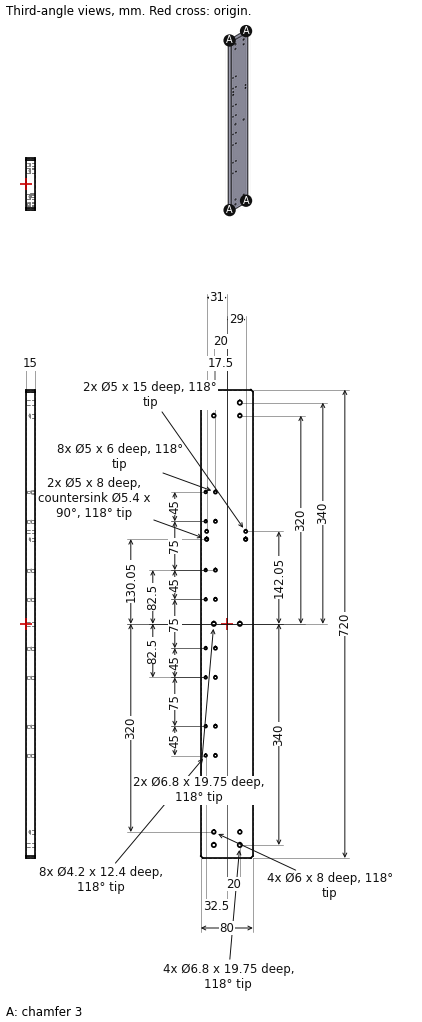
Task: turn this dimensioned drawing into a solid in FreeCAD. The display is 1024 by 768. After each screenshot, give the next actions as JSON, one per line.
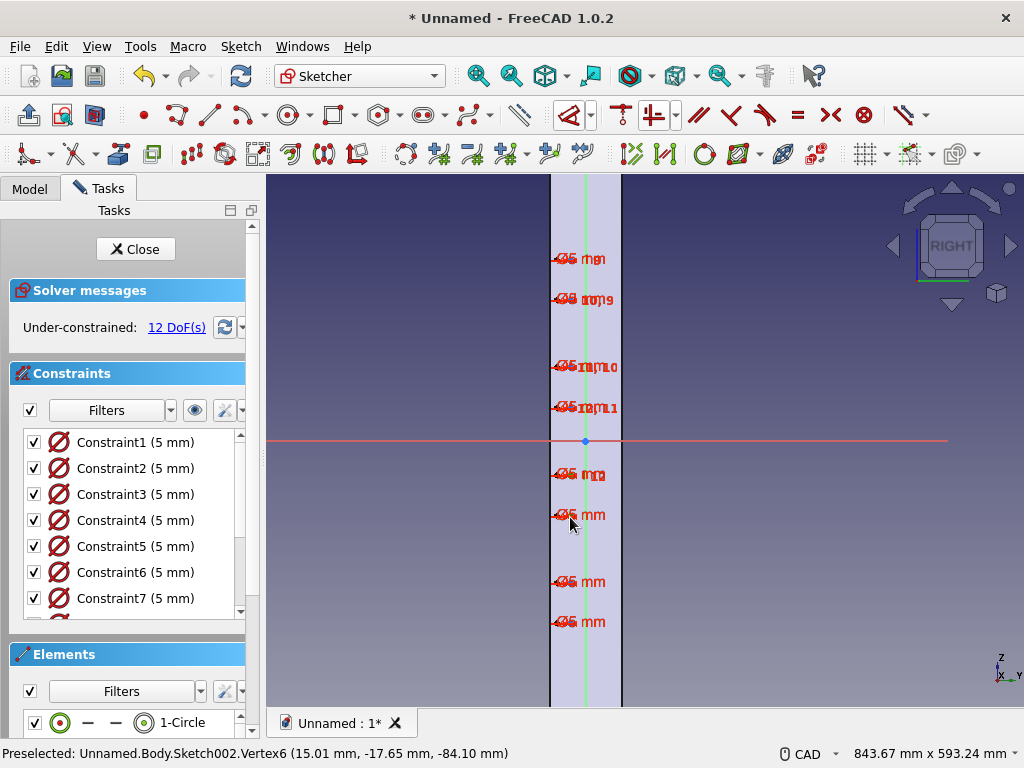
{"action": "left_click", "coordinate": [676, 116]}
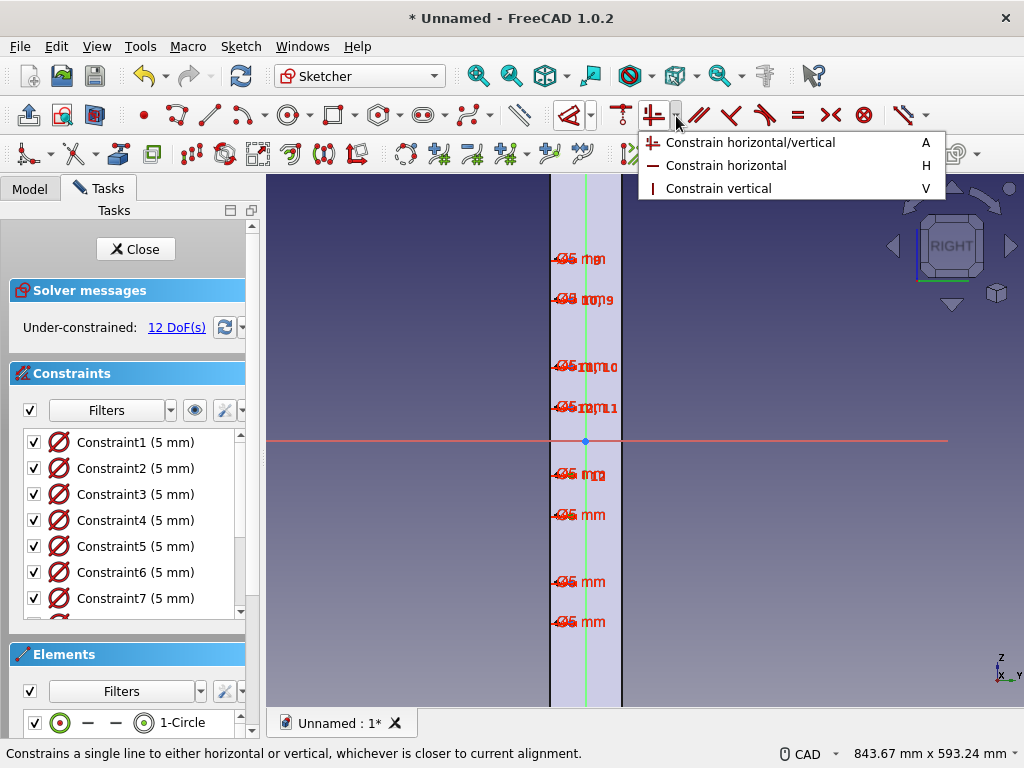
{"action": "left_click", "coordinate": [792, 188]}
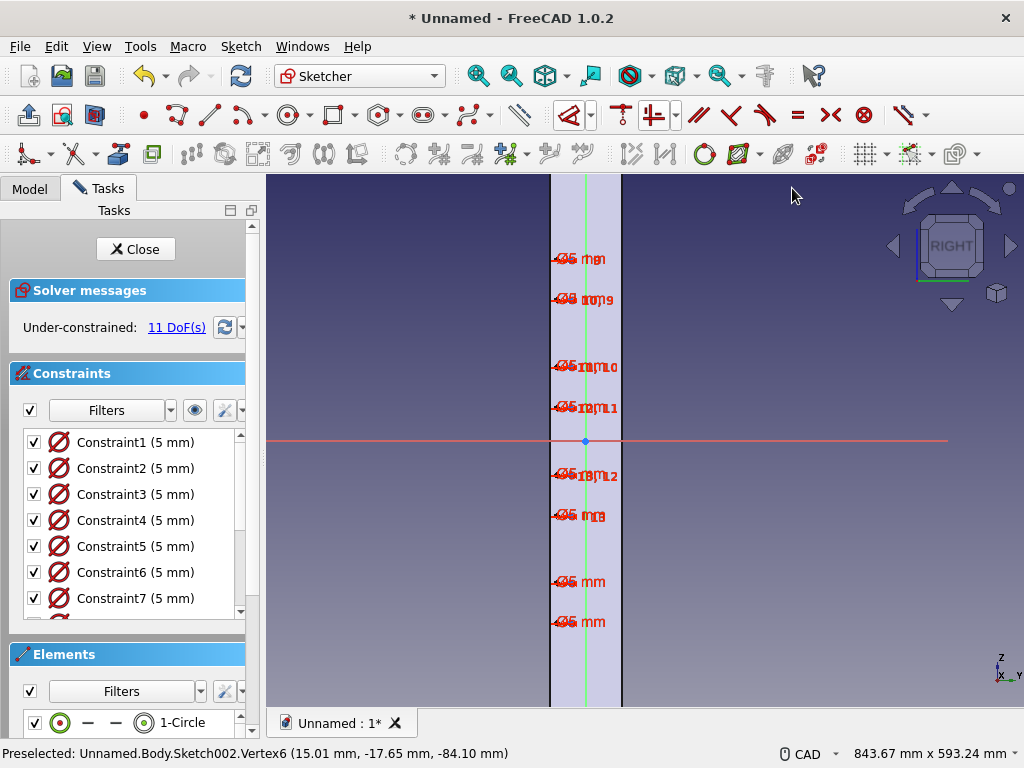
{"action": "left_click", "coordinate": [570, 517]}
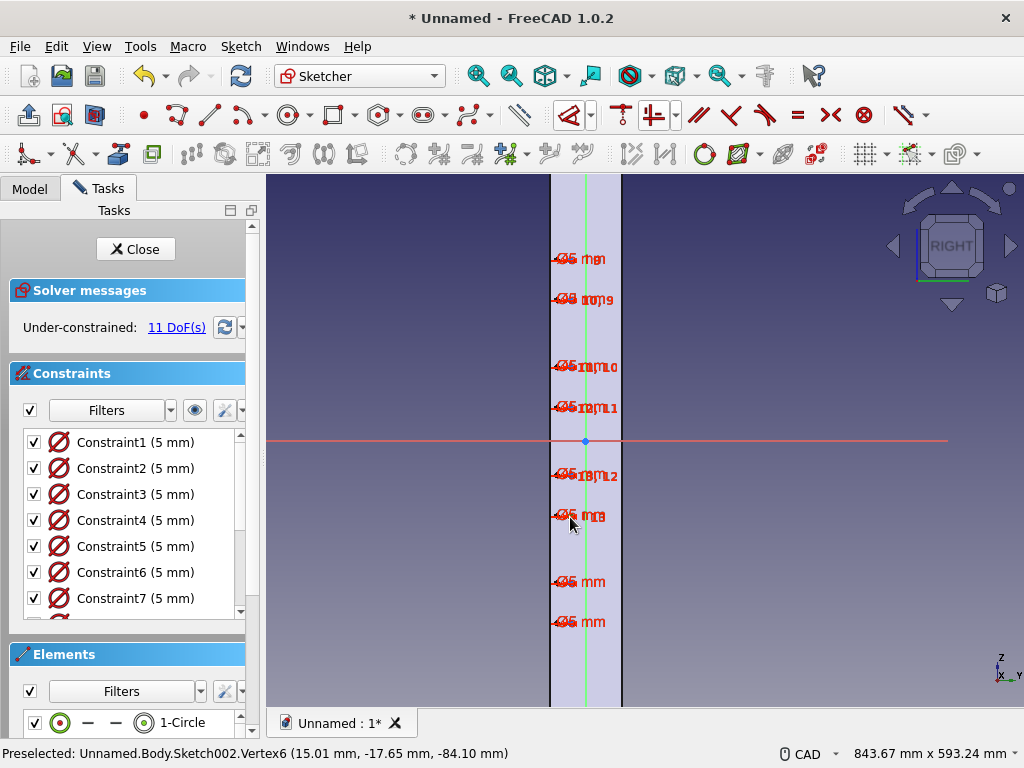
{"action": "left_click", "coordinate": [570, 584]}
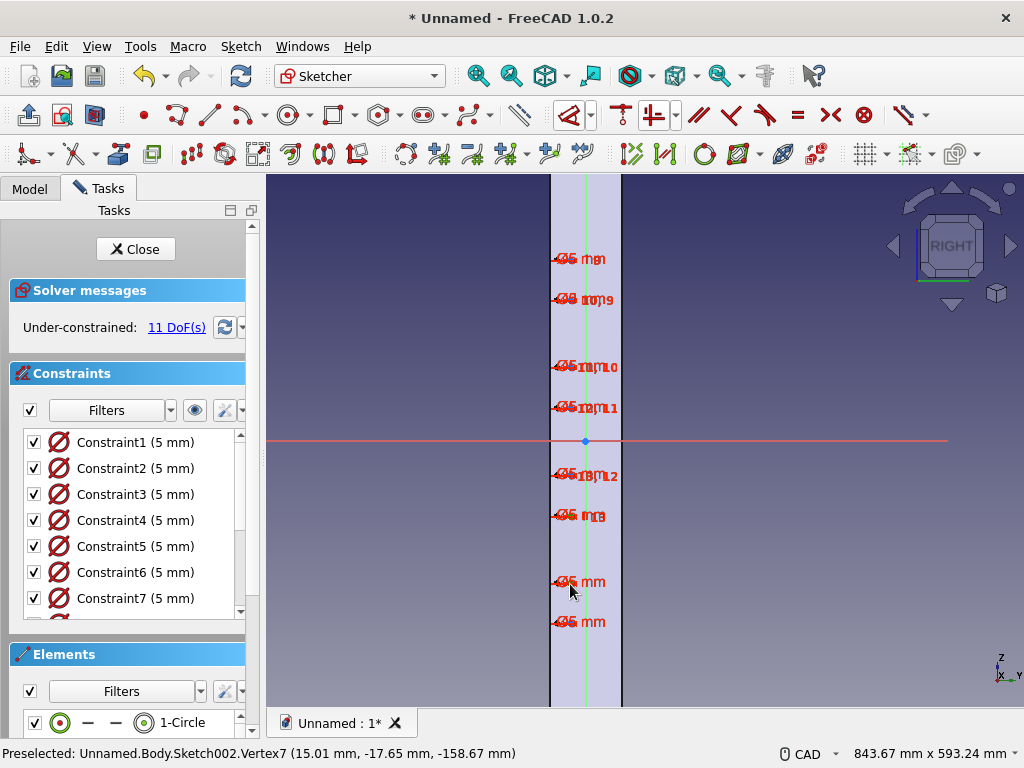
{"action": "left_click", "coordinate": [676, 116]}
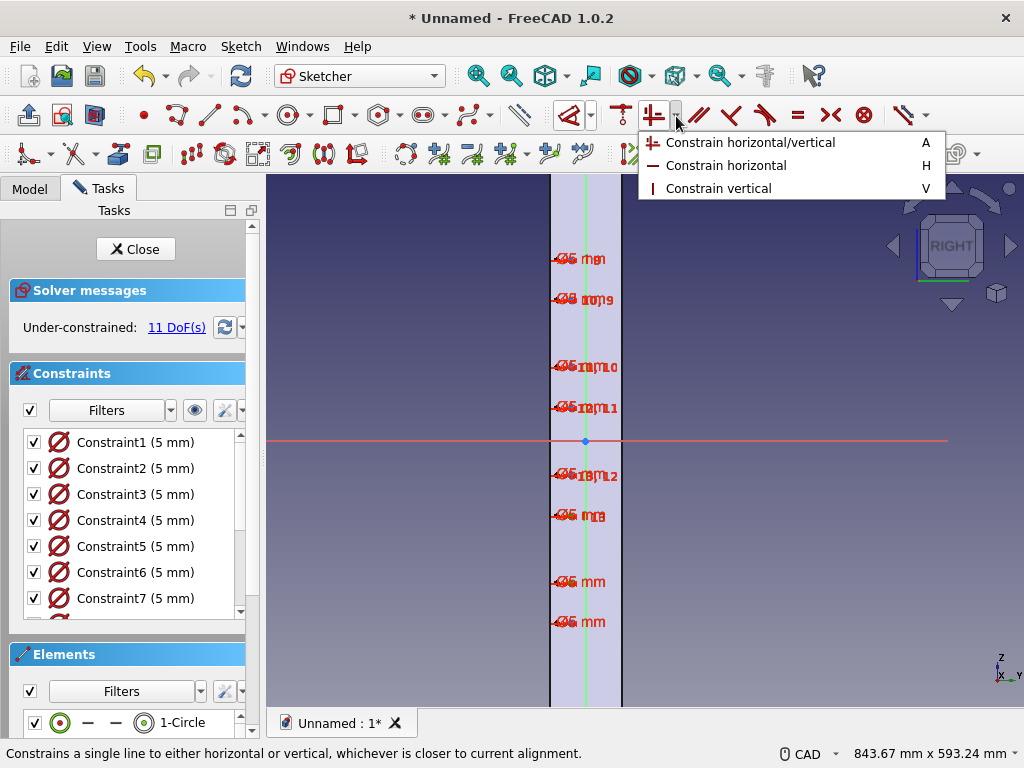
{"action": "left_click", "coordinate": [792, 188]}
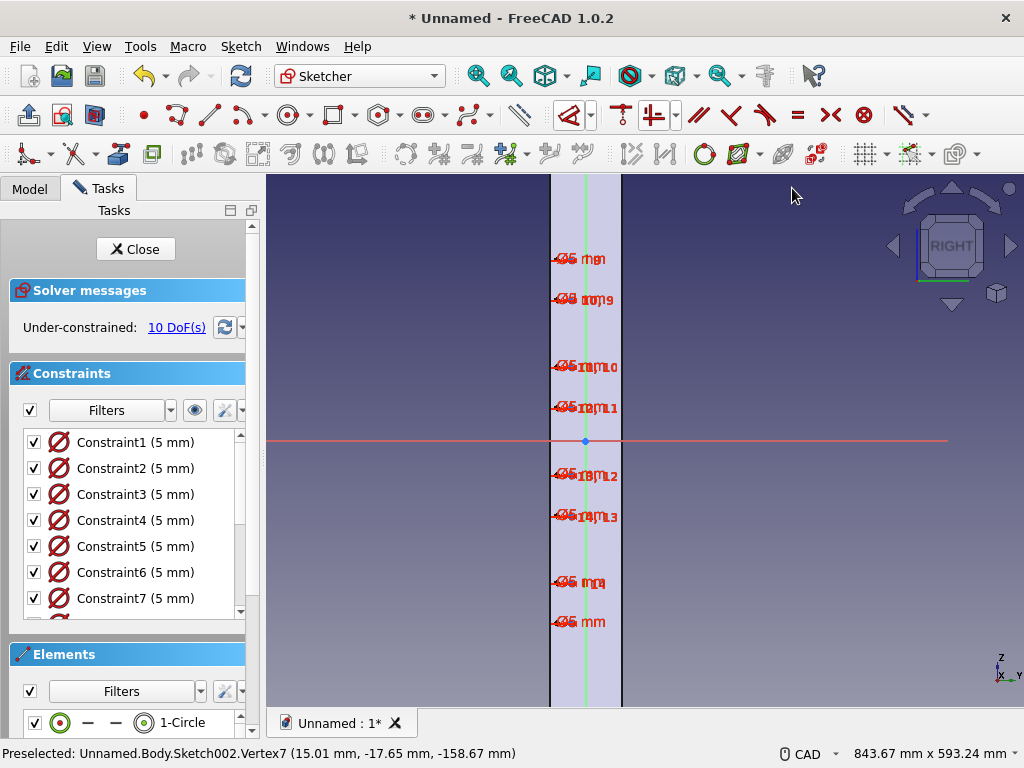
{"action": "left_click", "coordinate": [570, 584]}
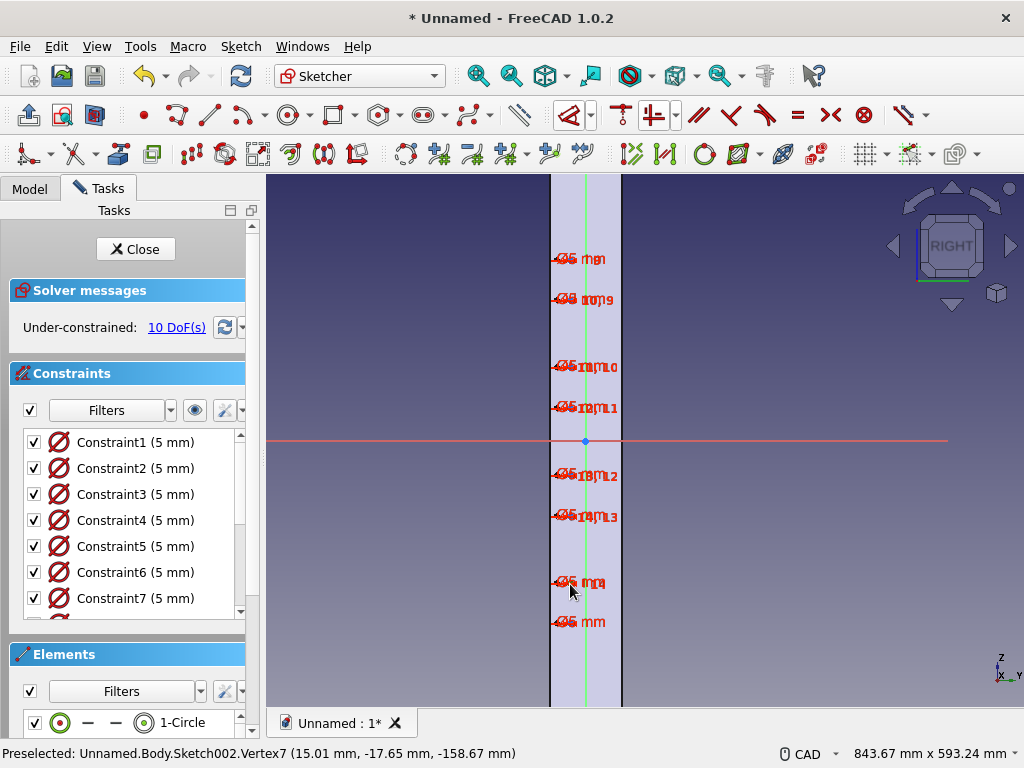
{"action": "left_click", "coordinate": [570, 624]}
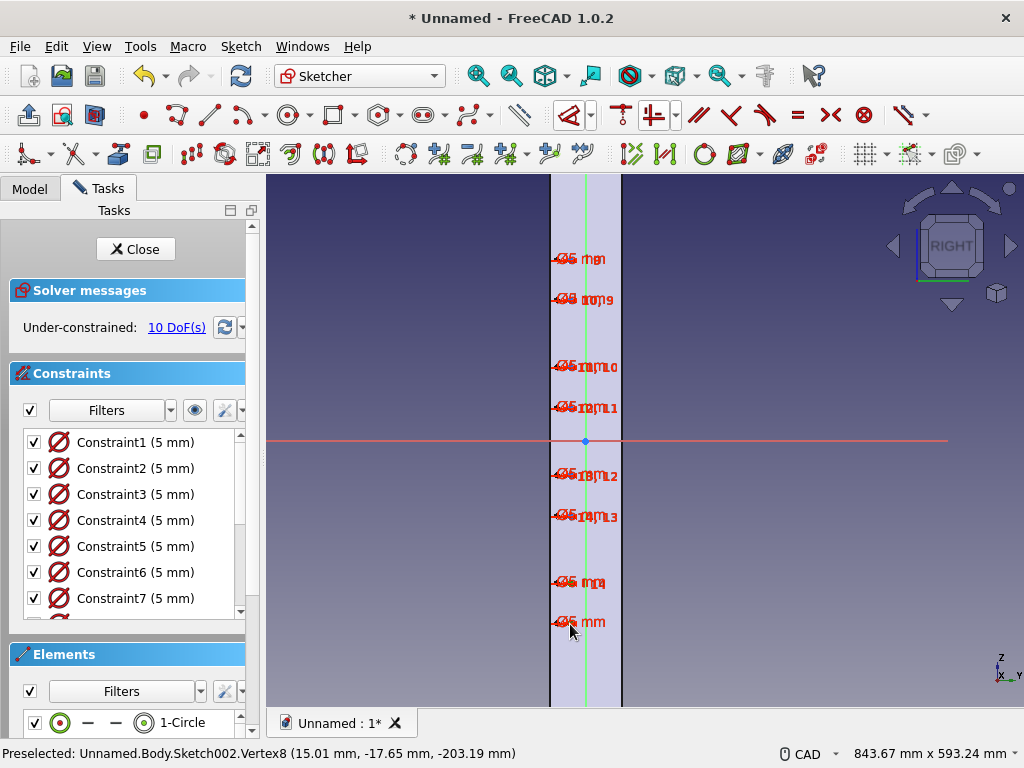
{"action": "key", "text": "v"}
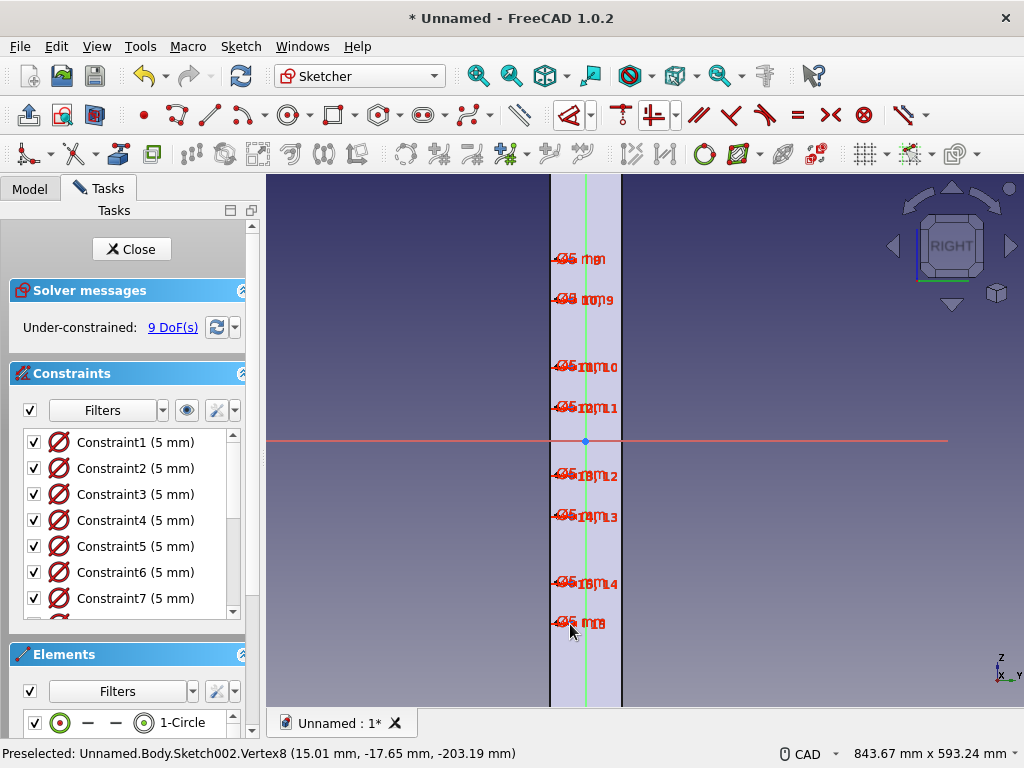
{"action": "left_click", "coordinate": [570, 261]}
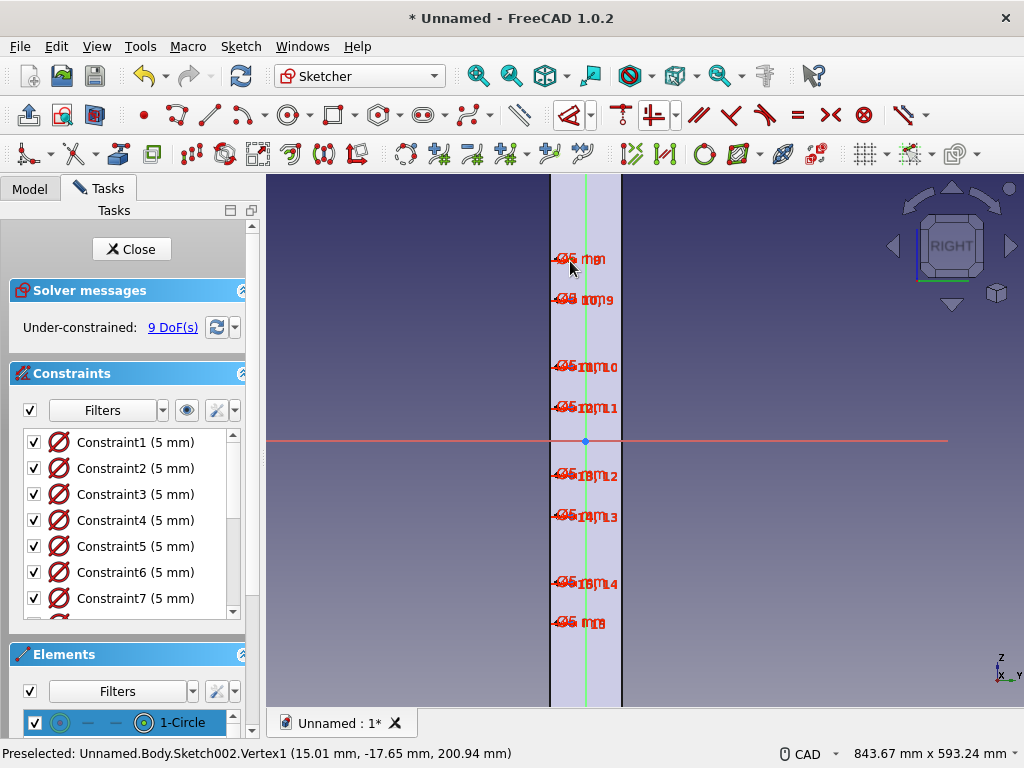
{"action": "left_click", "coordinate": [570, 301]}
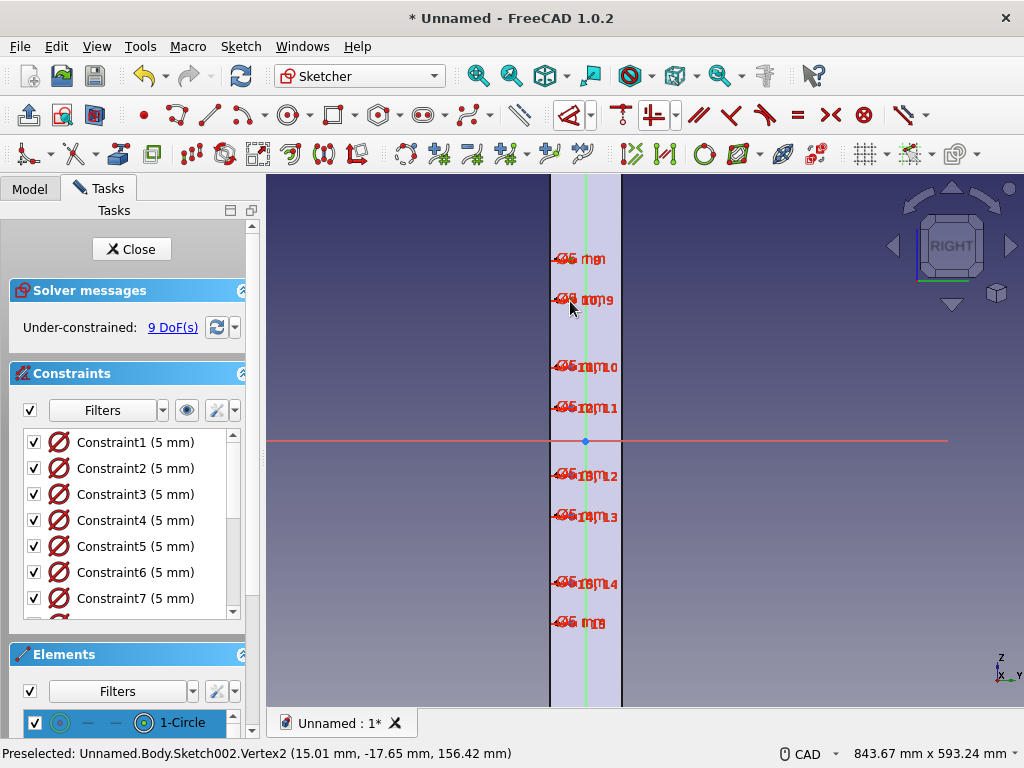
{"action": "left_click", "coordinate": [590, 116]}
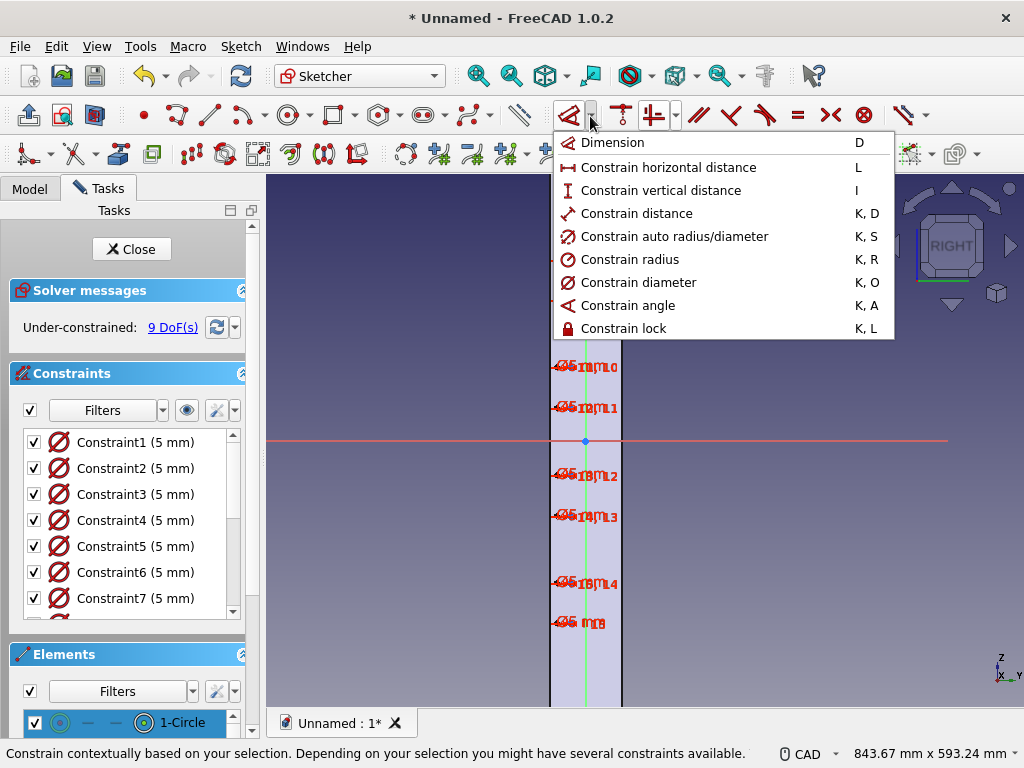
{"action": "left_click", "coordinate": [724, 190]}